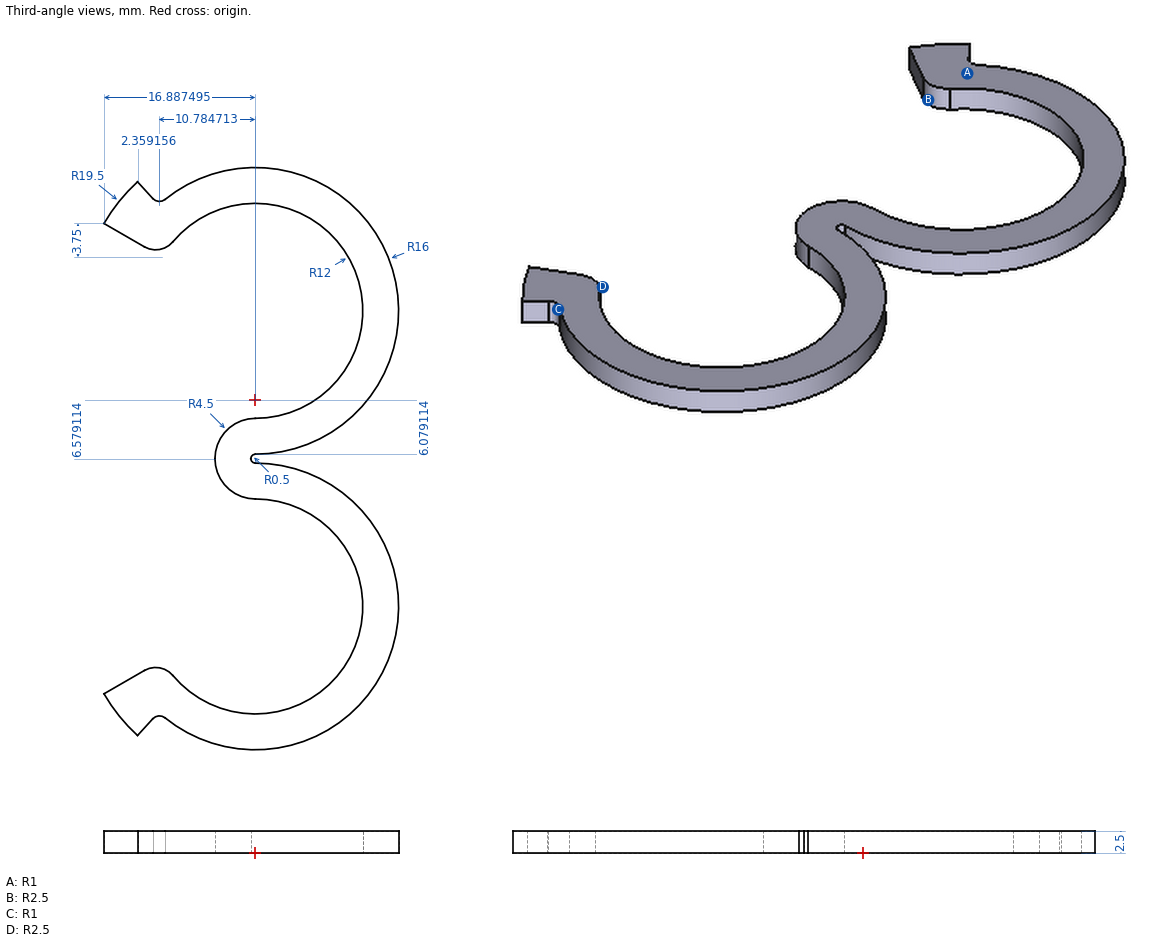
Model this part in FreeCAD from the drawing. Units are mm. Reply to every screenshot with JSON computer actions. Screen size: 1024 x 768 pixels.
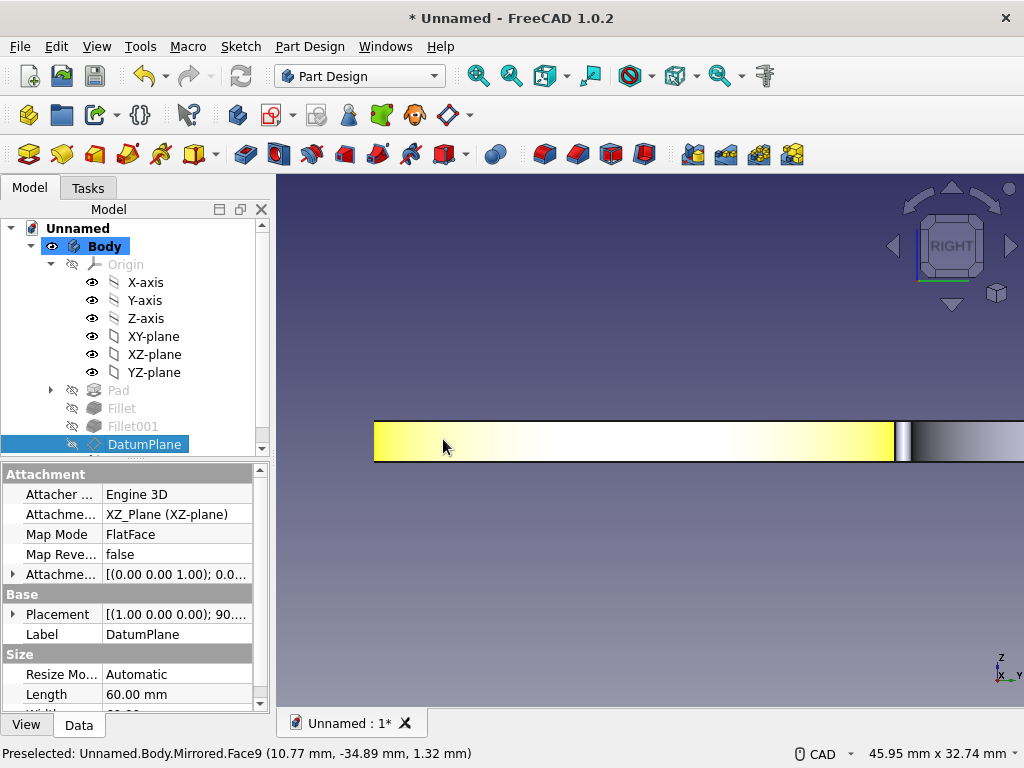
{"action": "left_click", "coordinate": [479, 76]}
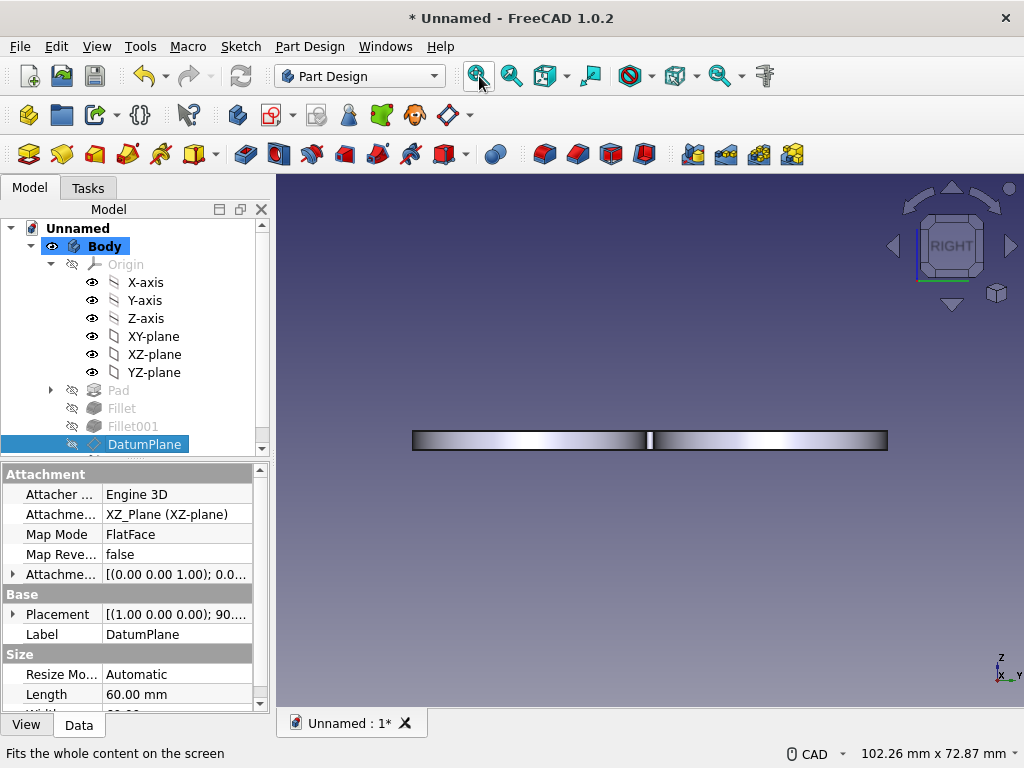
{"action": "key", "text": "5"}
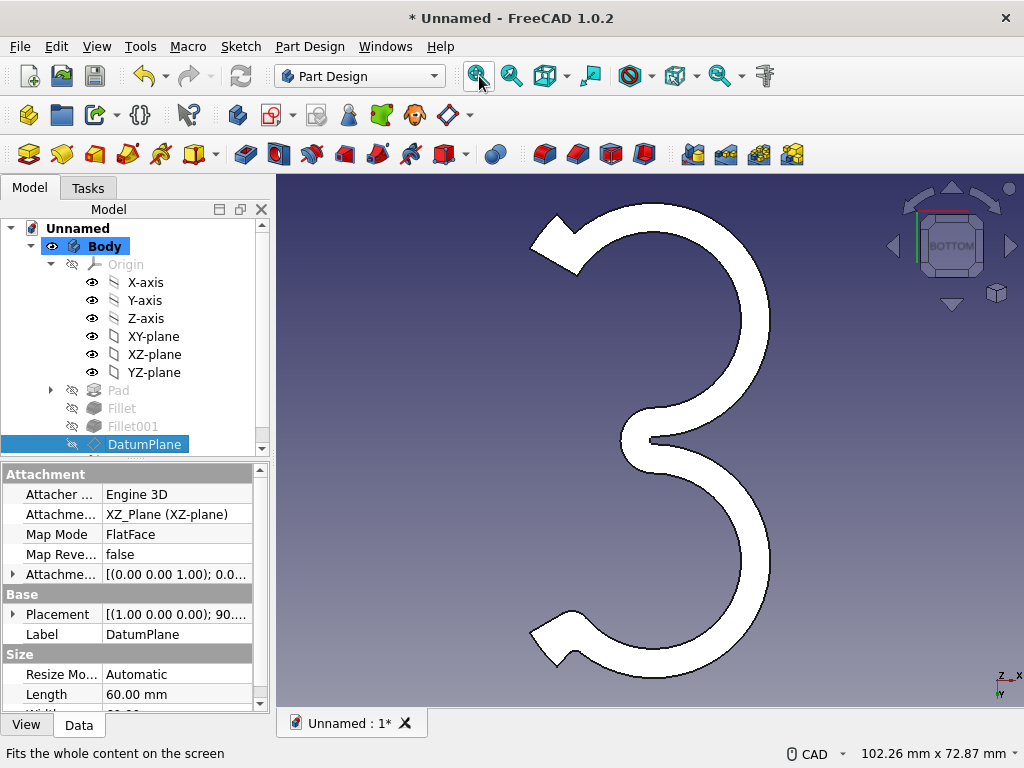
{"action": "scroll", "coordinate": [574, 232], "scroll_direction": "up", "scroll_amount": 4}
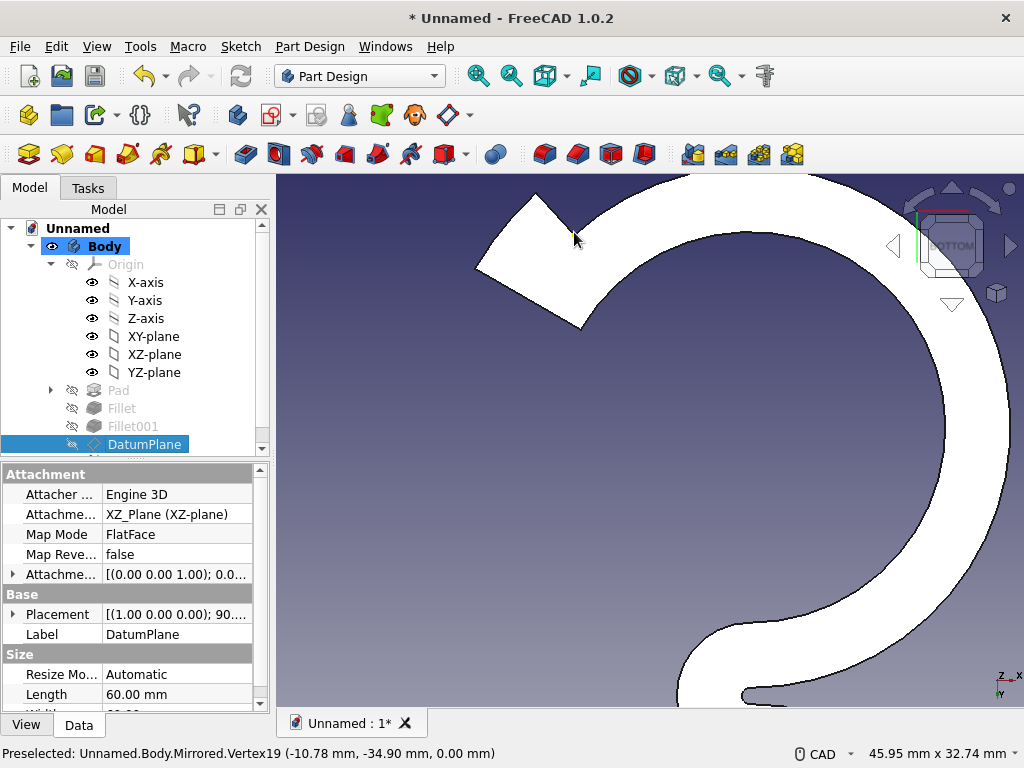
{"action": "left_click", "coordinate": [479, 76]}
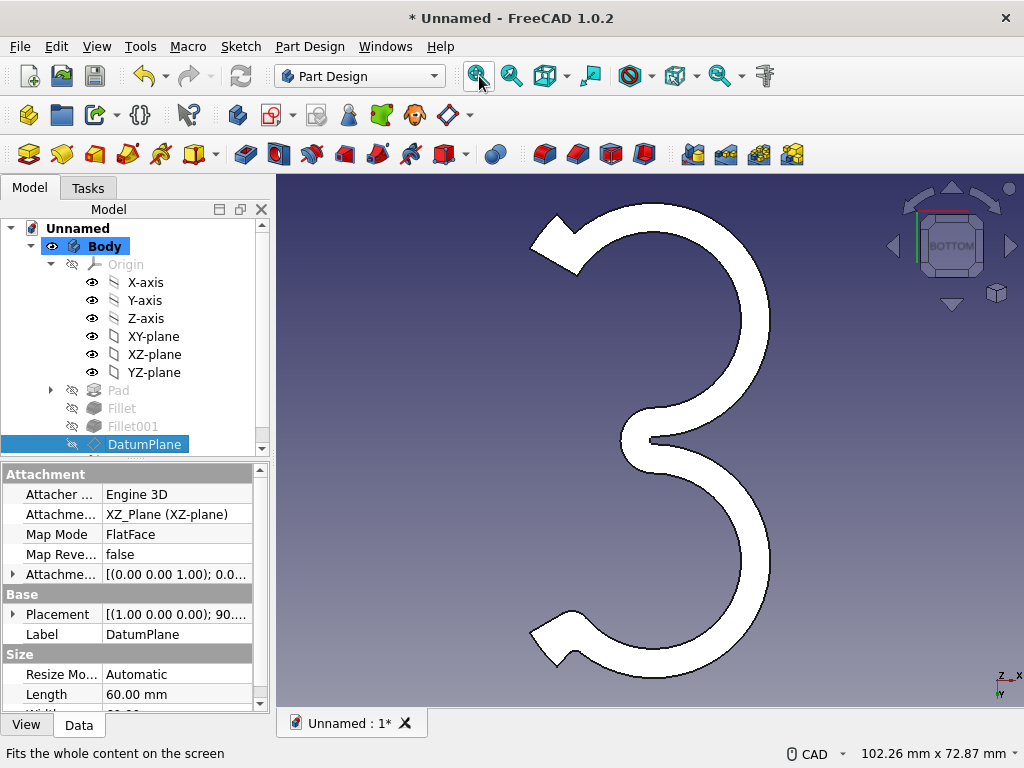
{"action": "key", "text": "4"}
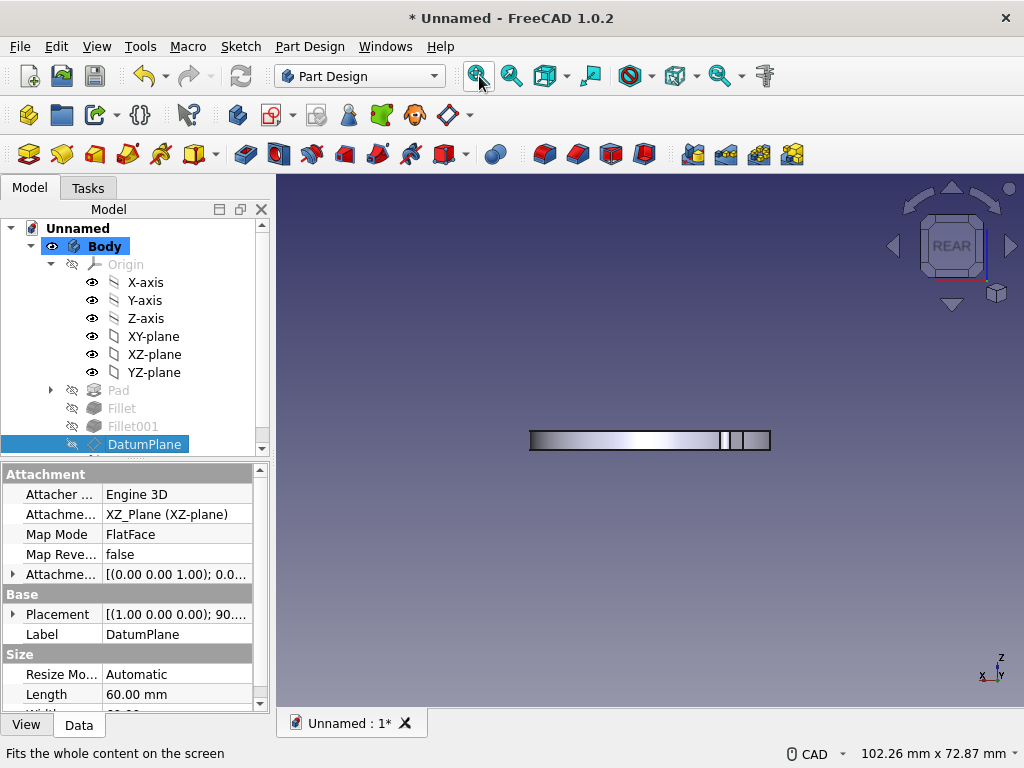
{"action": "left_click", "coordinate": [479, 76]}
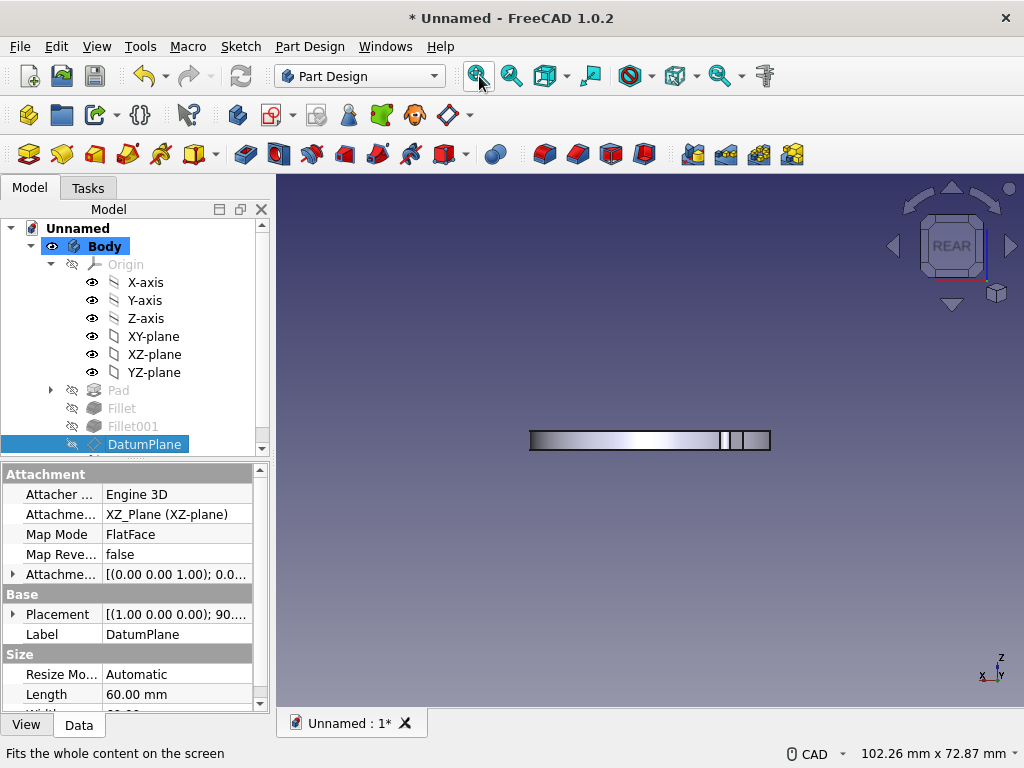
{"action": "scroll", "coordinate": [726, 440], "scroll_direction": "up", "scroll_amount": 4}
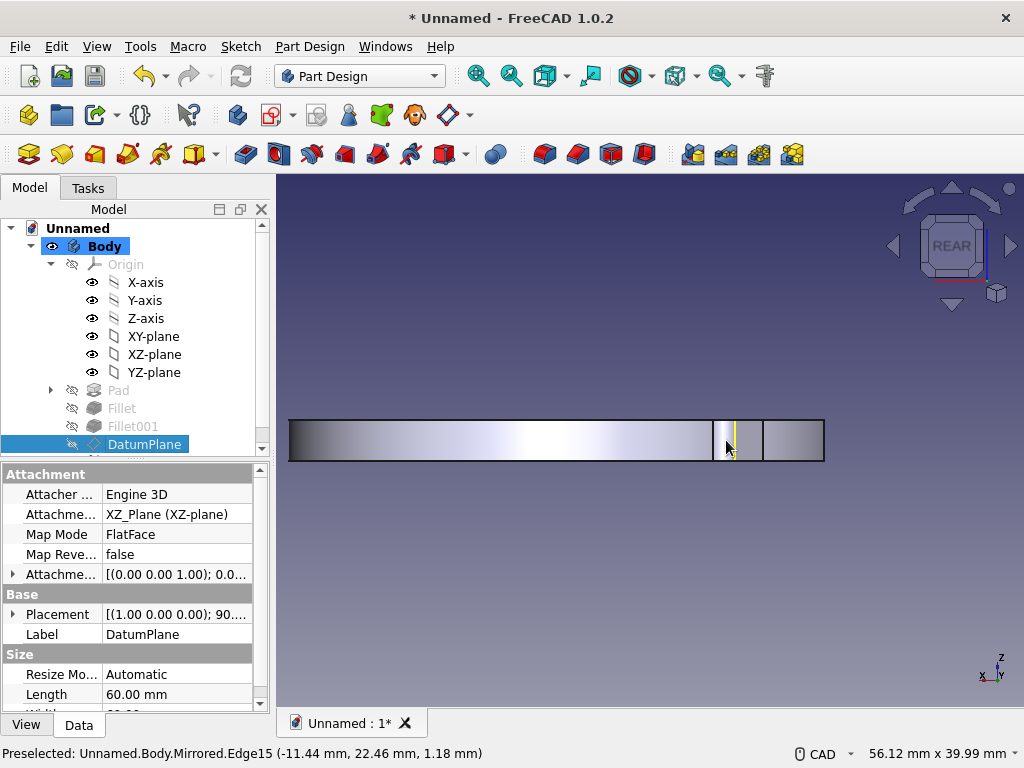
{"action": "left_click", "coordinate": [479, 76]}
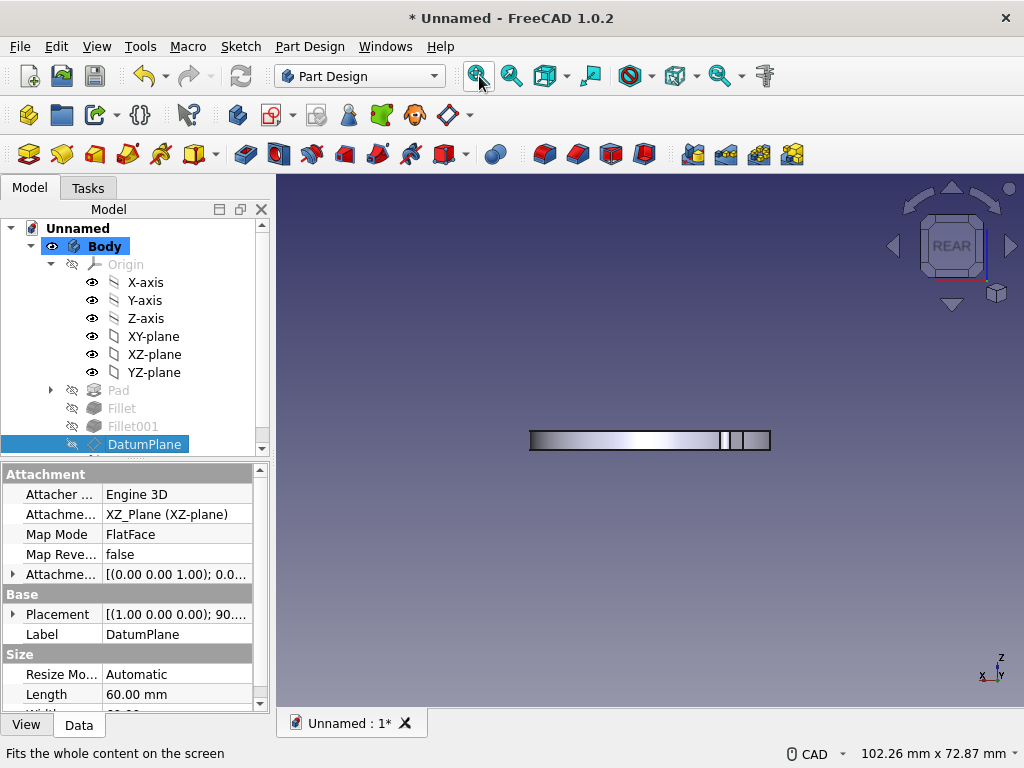
{"action": "key", "text": "6"}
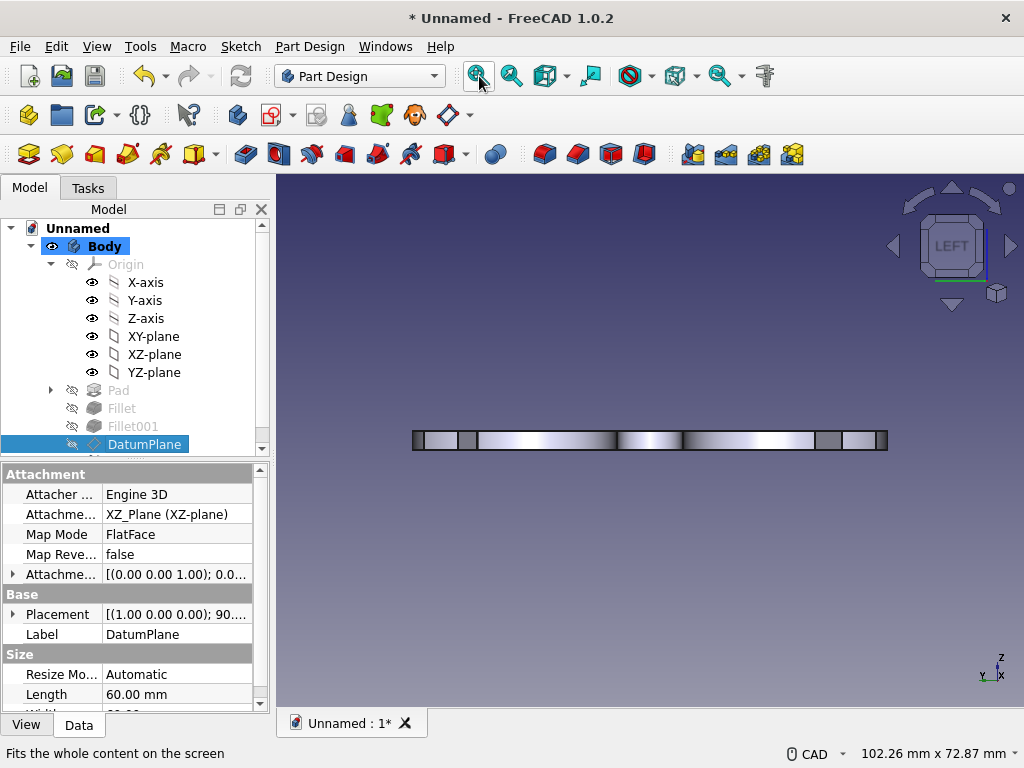
{"action": "scroll", "coordinate": [857, 439], "scroll_direction": "up", "scroll_amount": 4}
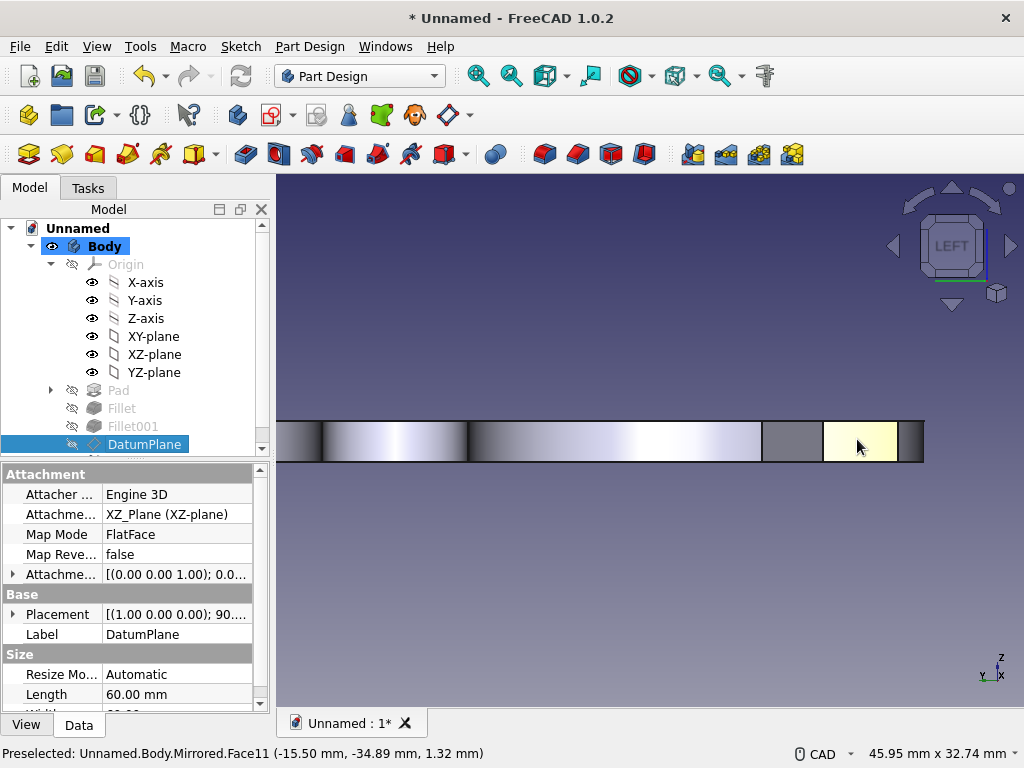
{"action": "left_click", "coordinate": [479, 76]}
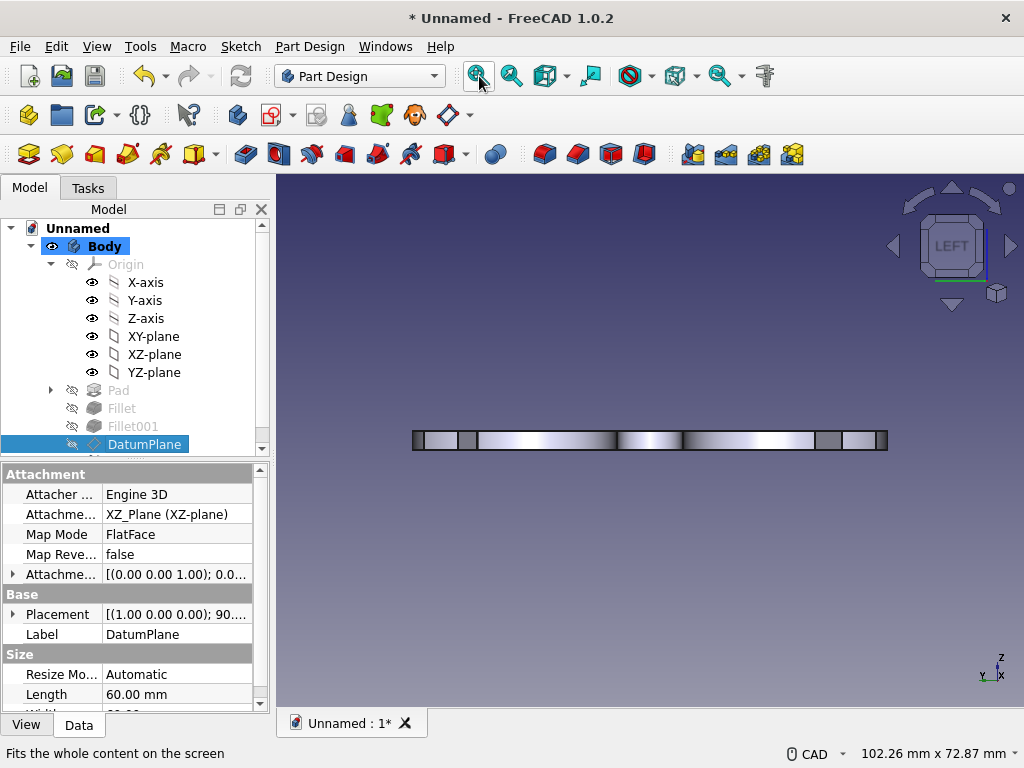
{"action": "key", "text": "v 3"}